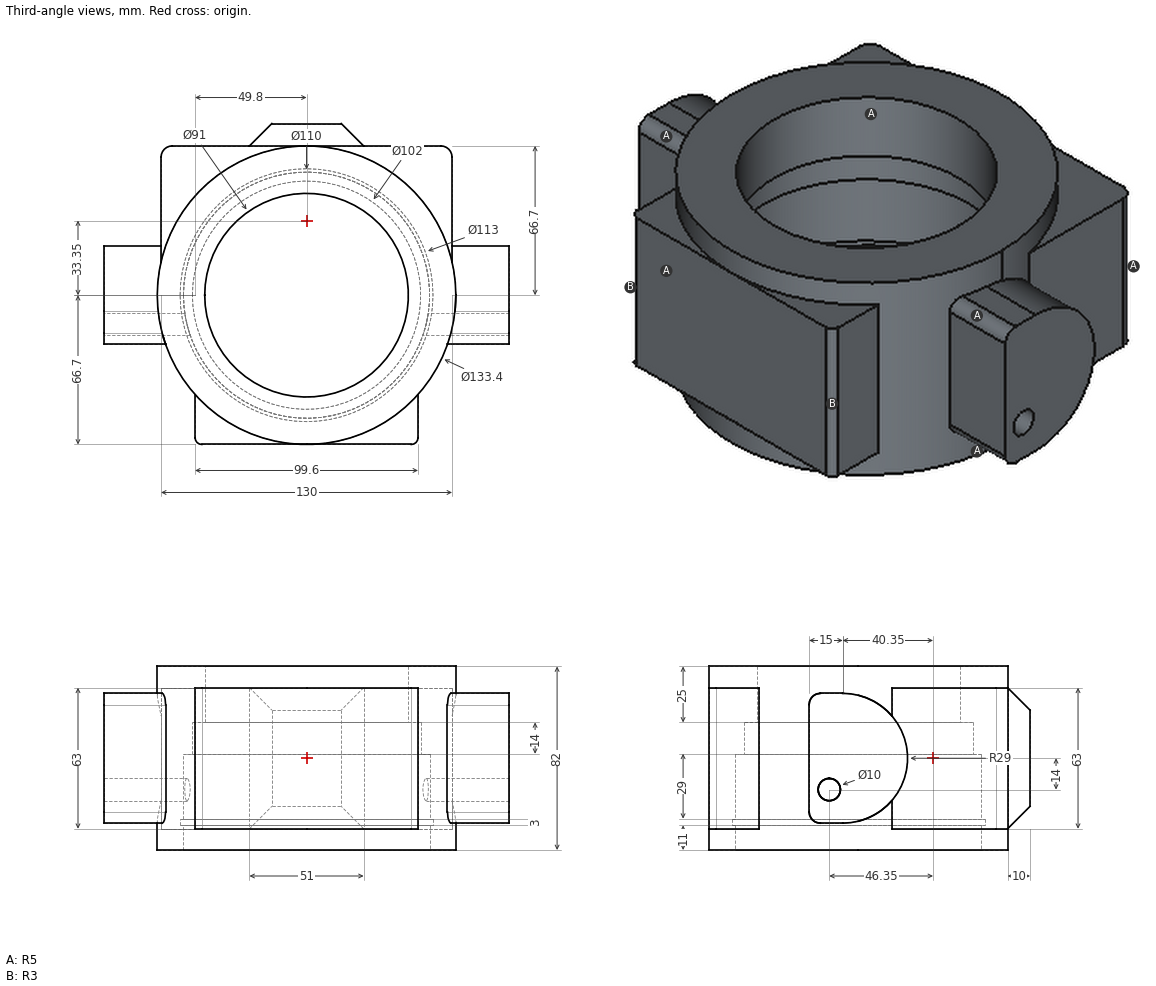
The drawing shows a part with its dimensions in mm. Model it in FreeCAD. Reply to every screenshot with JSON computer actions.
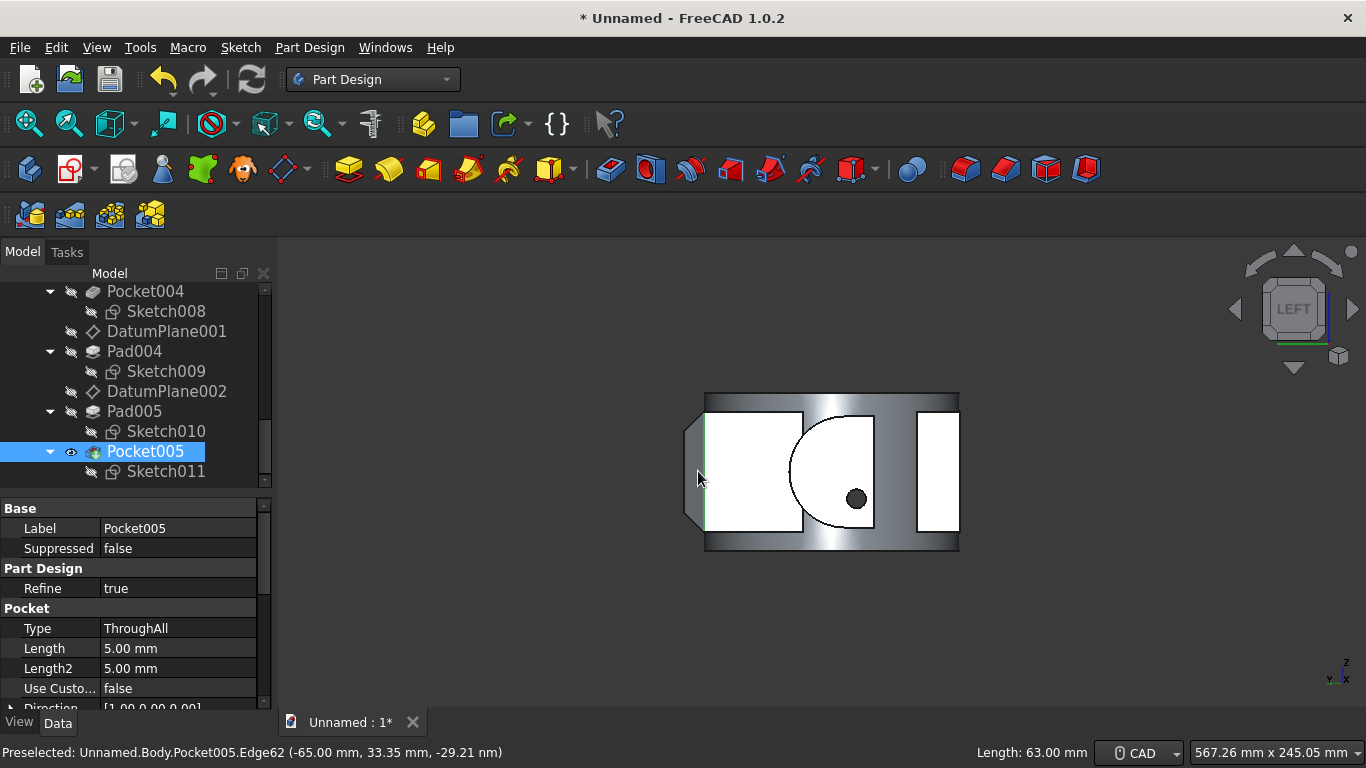
{"action": "key", "text": "0"}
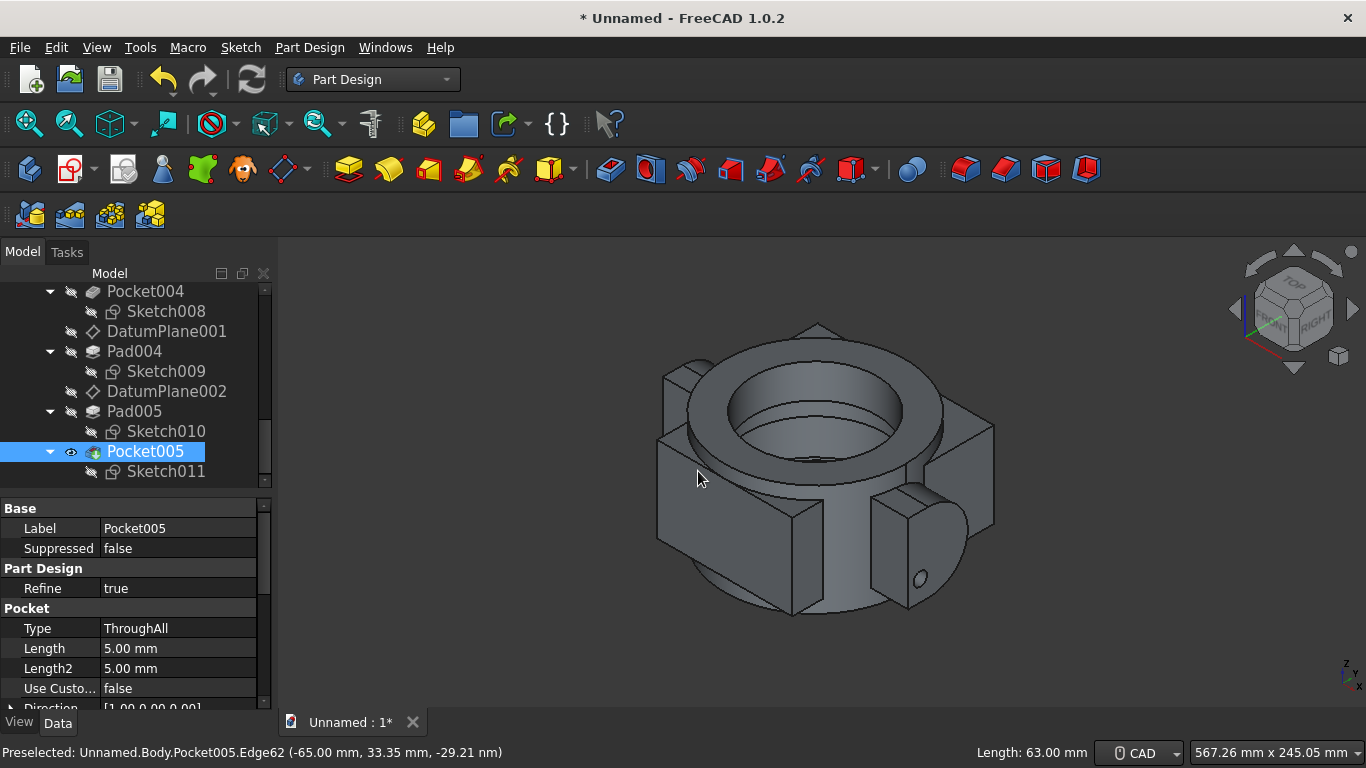
{"action": "left_click", "coordinate": [681, 387], "text": "ctrl"}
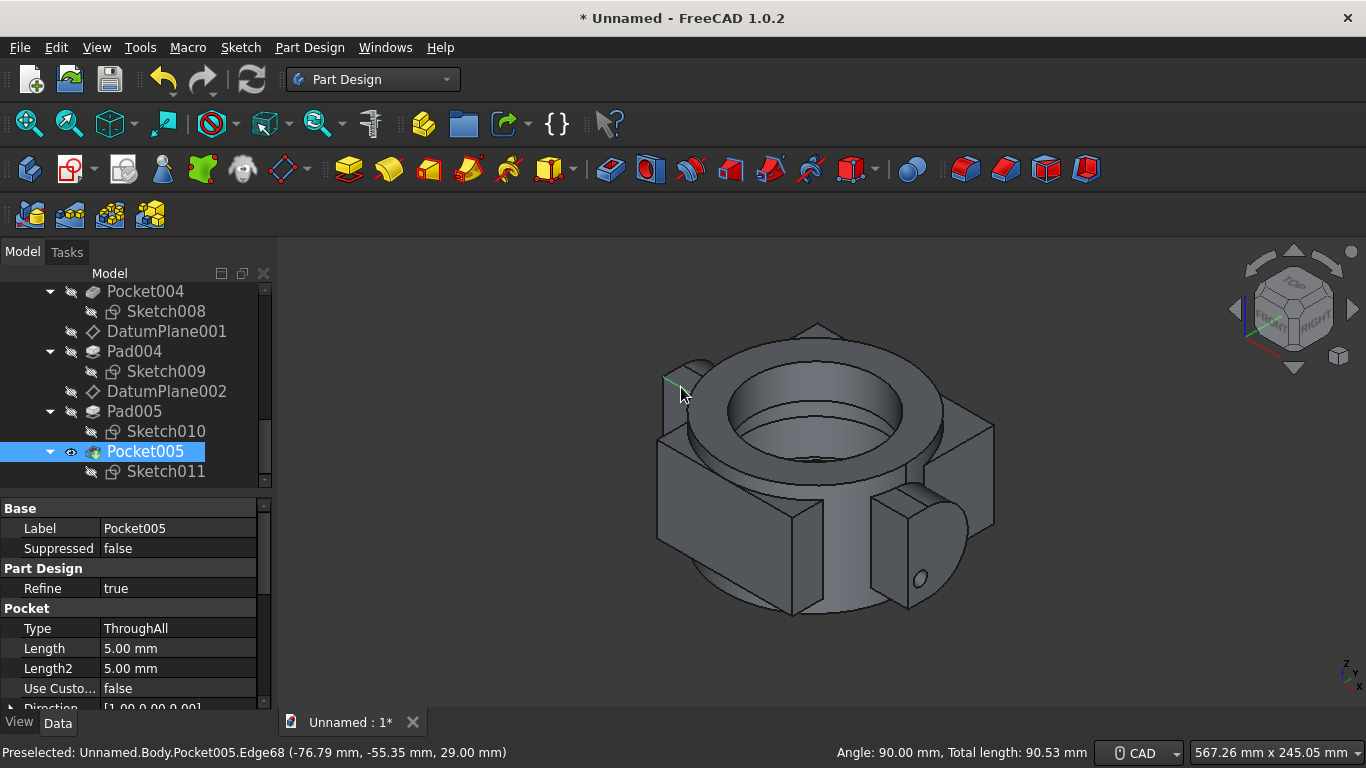
{"action": "left_click", "coordinate": [889, 507], "text": "ctrl"}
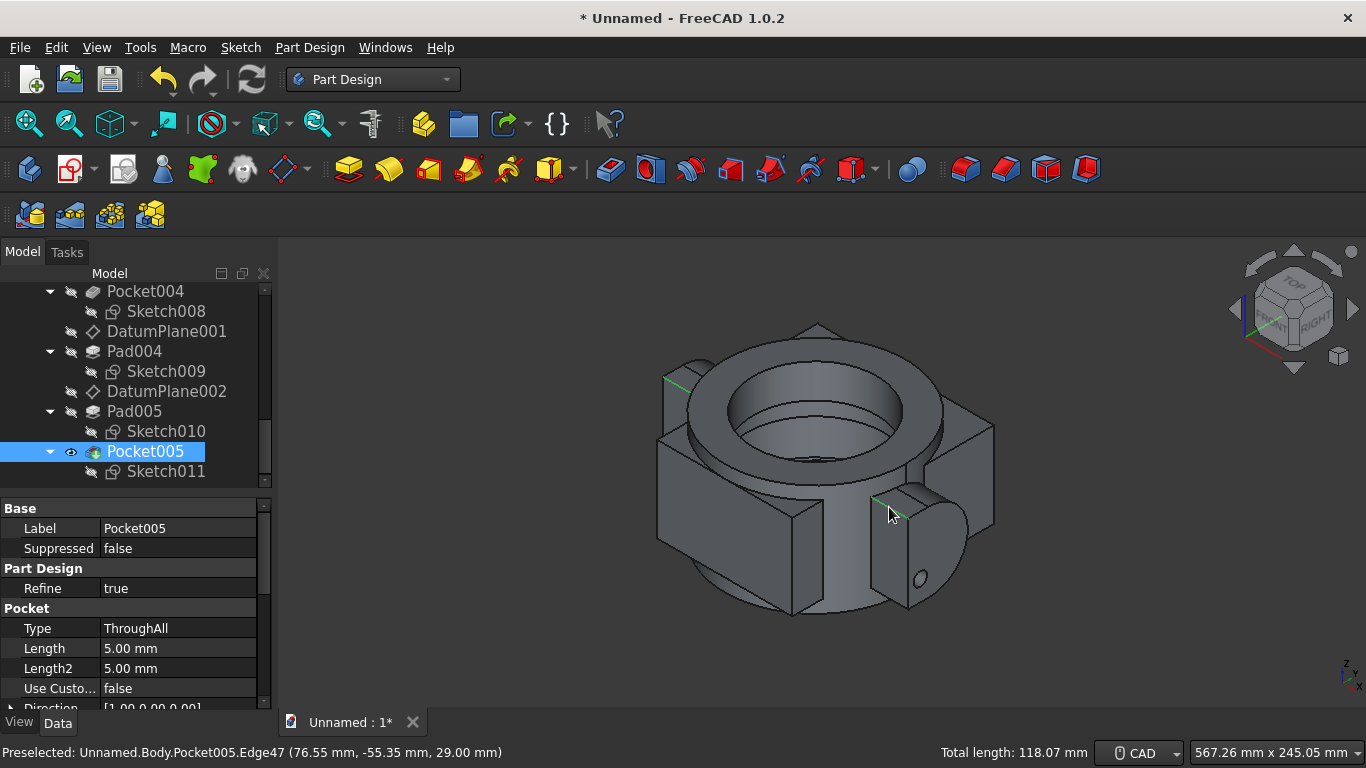
{"action": "key", "text": "2"}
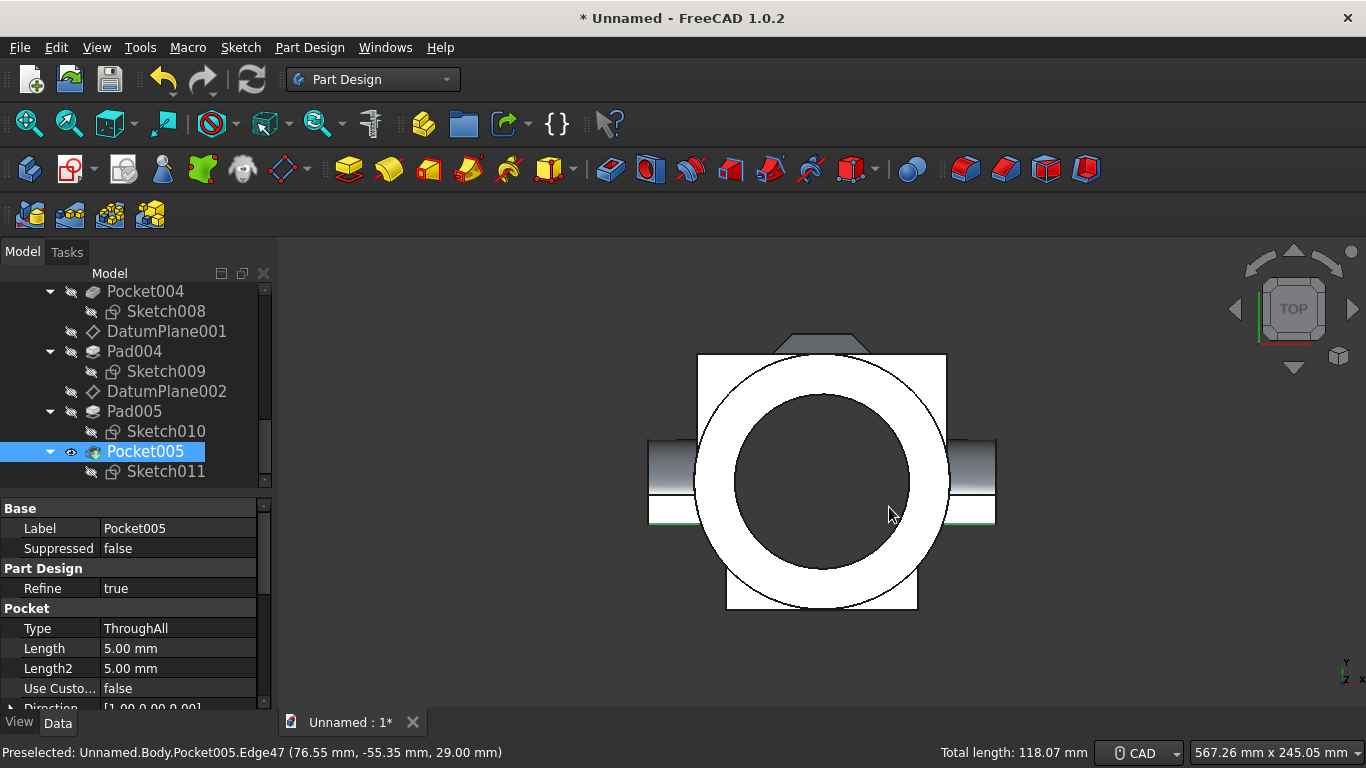
{"action": "key", "text": "1"}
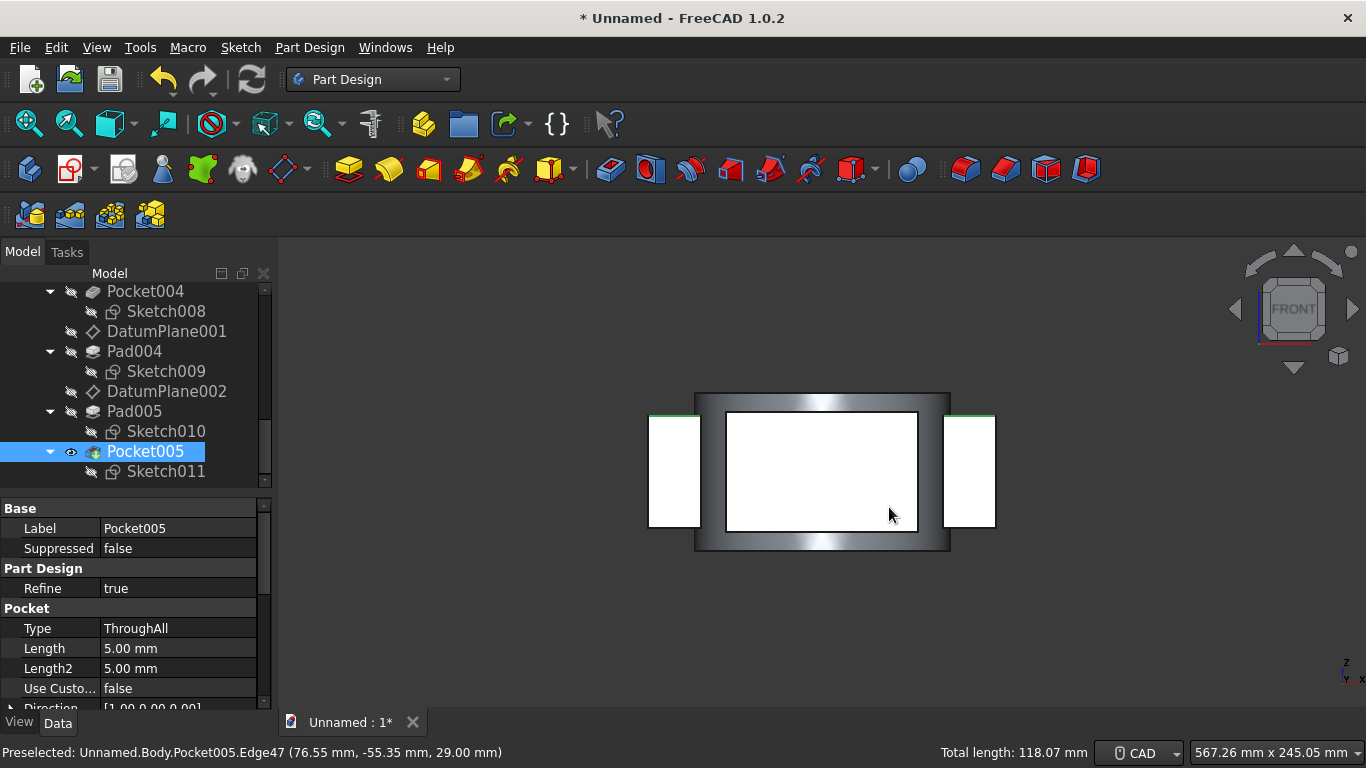
{"action": "key", "text": "v f"}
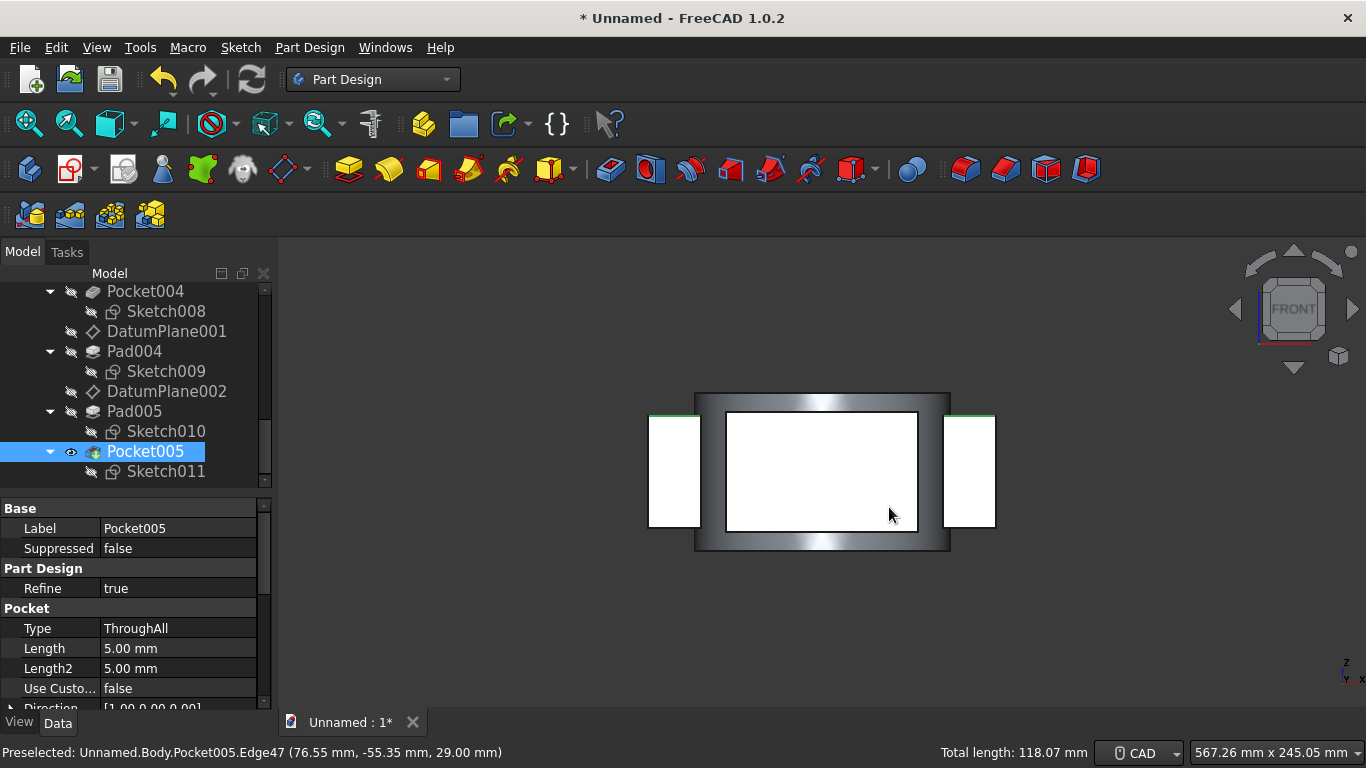
{"action": "left_click", "coordinate": [675, 527], "text": "ctrl"}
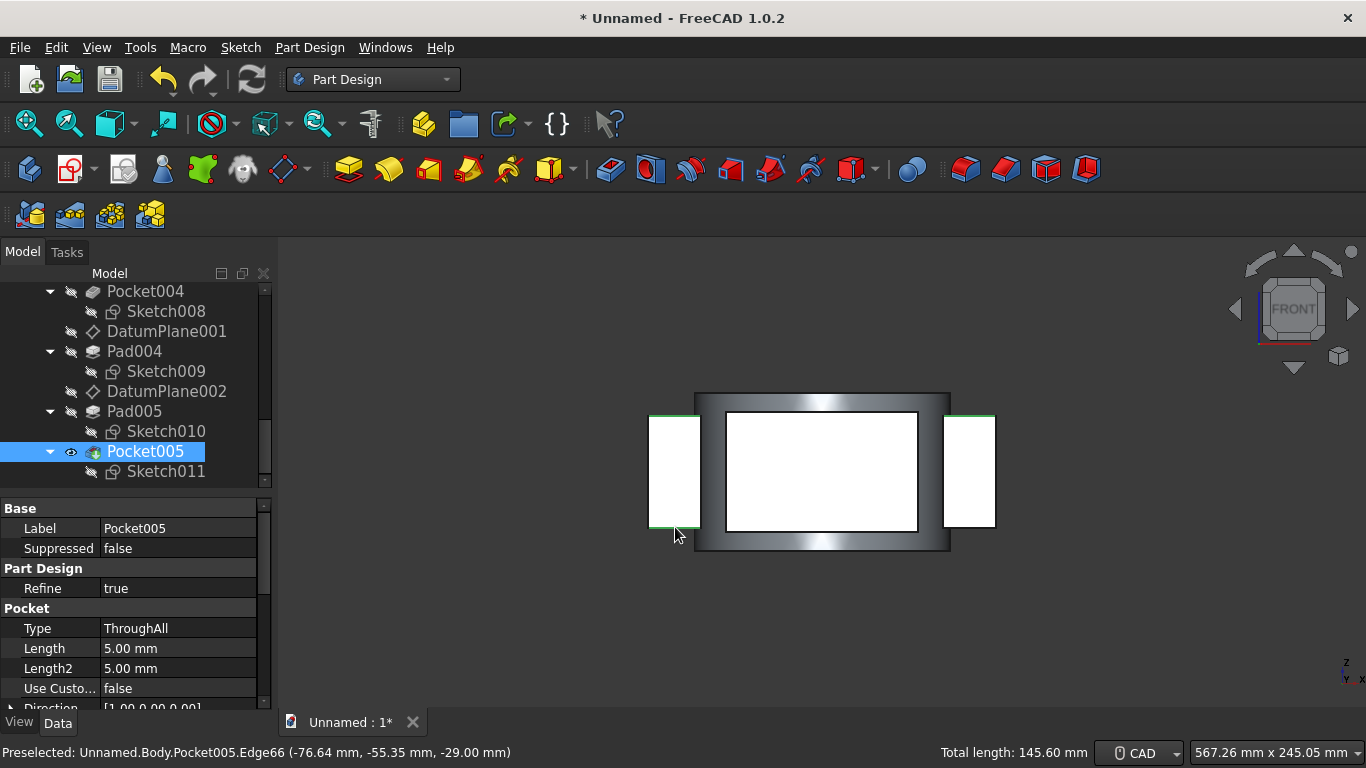
{"action": "left_click", "coordinate": [969, 527], "text": "ctrl"}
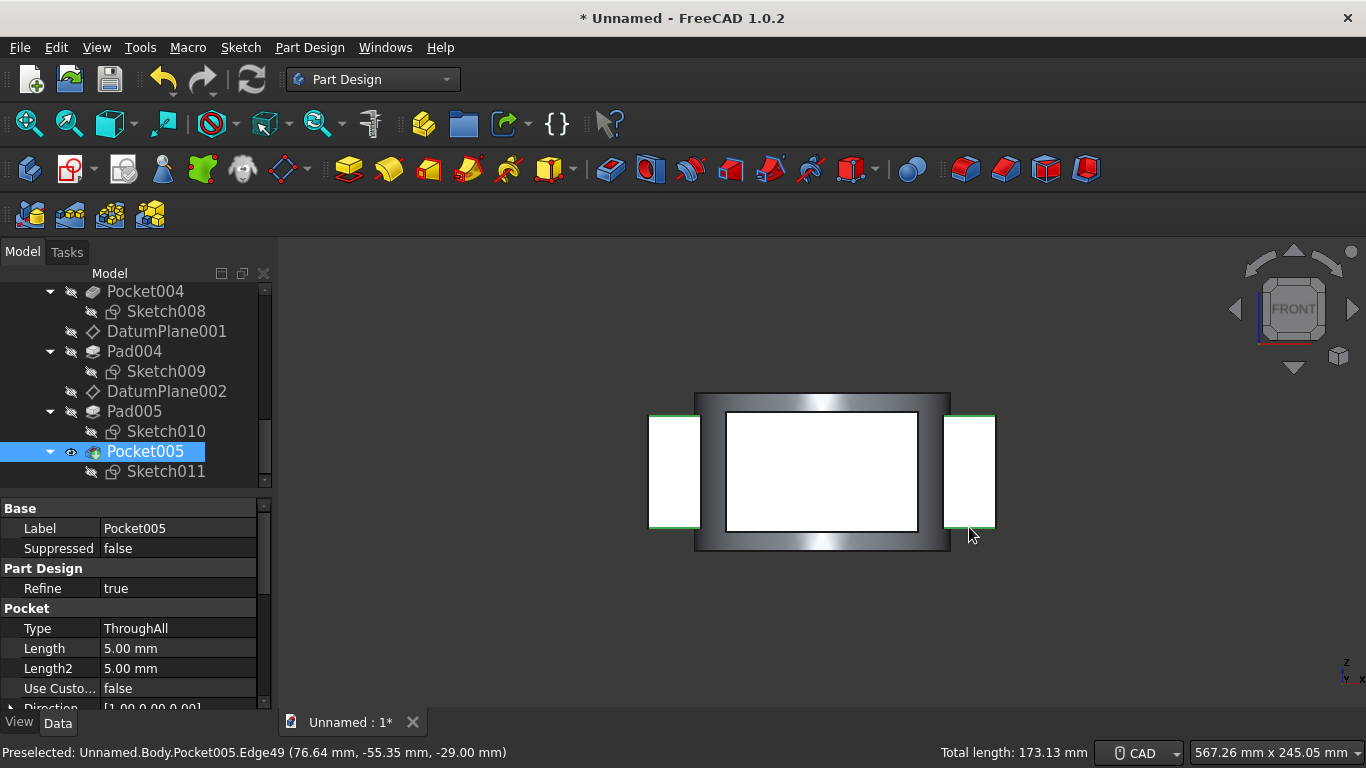
{"action": "key", "text": "3"}